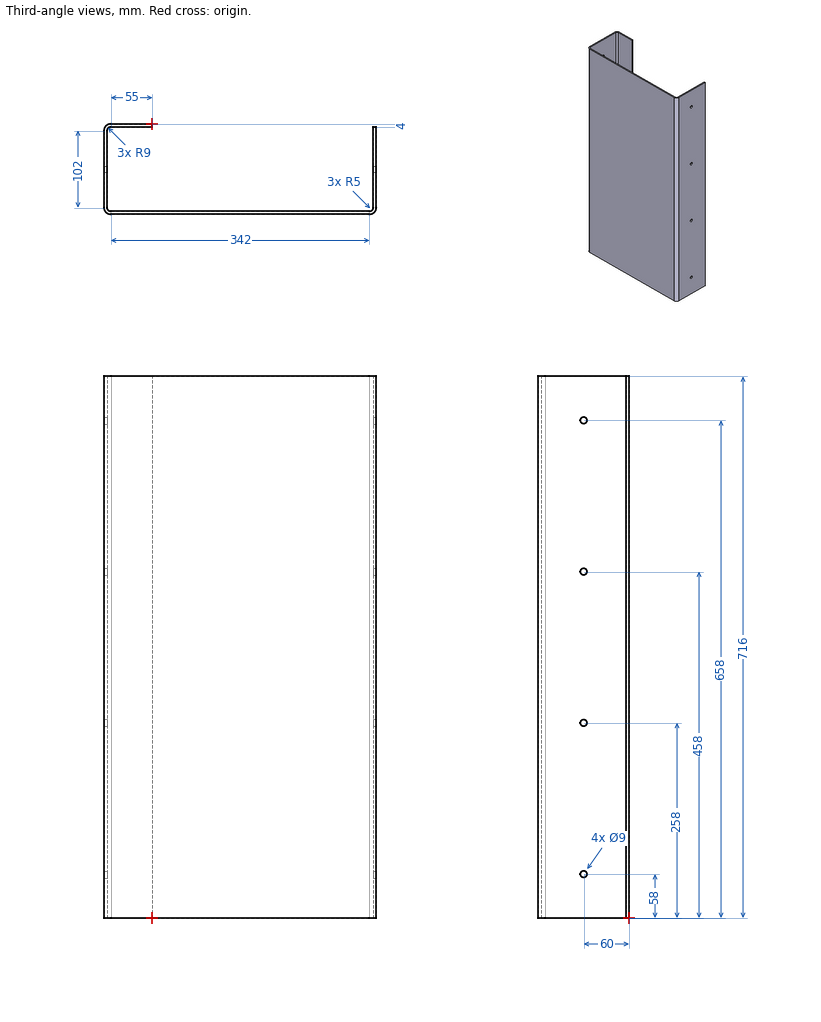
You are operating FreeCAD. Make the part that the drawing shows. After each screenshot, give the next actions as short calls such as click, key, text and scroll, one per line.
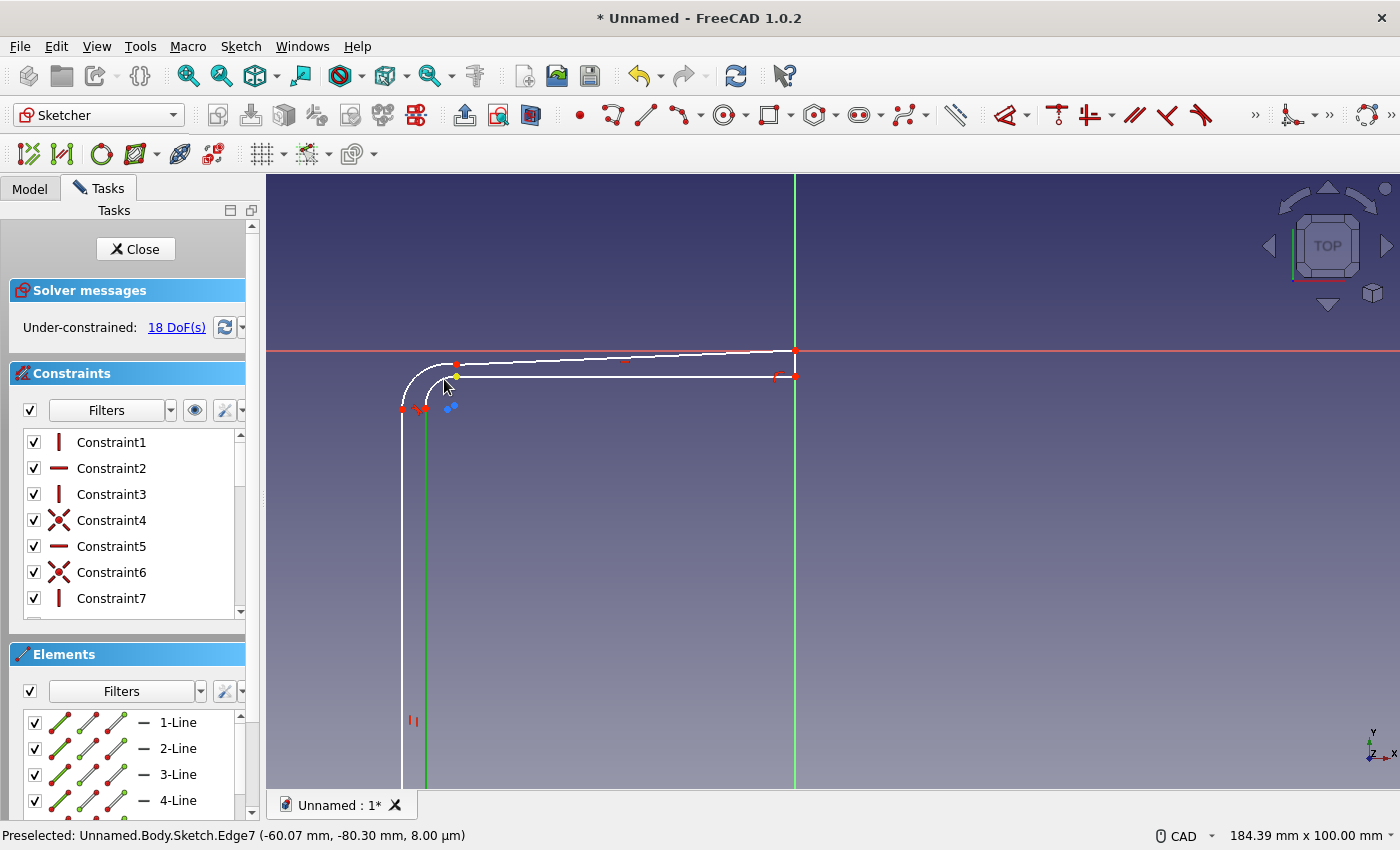
click(442, 380)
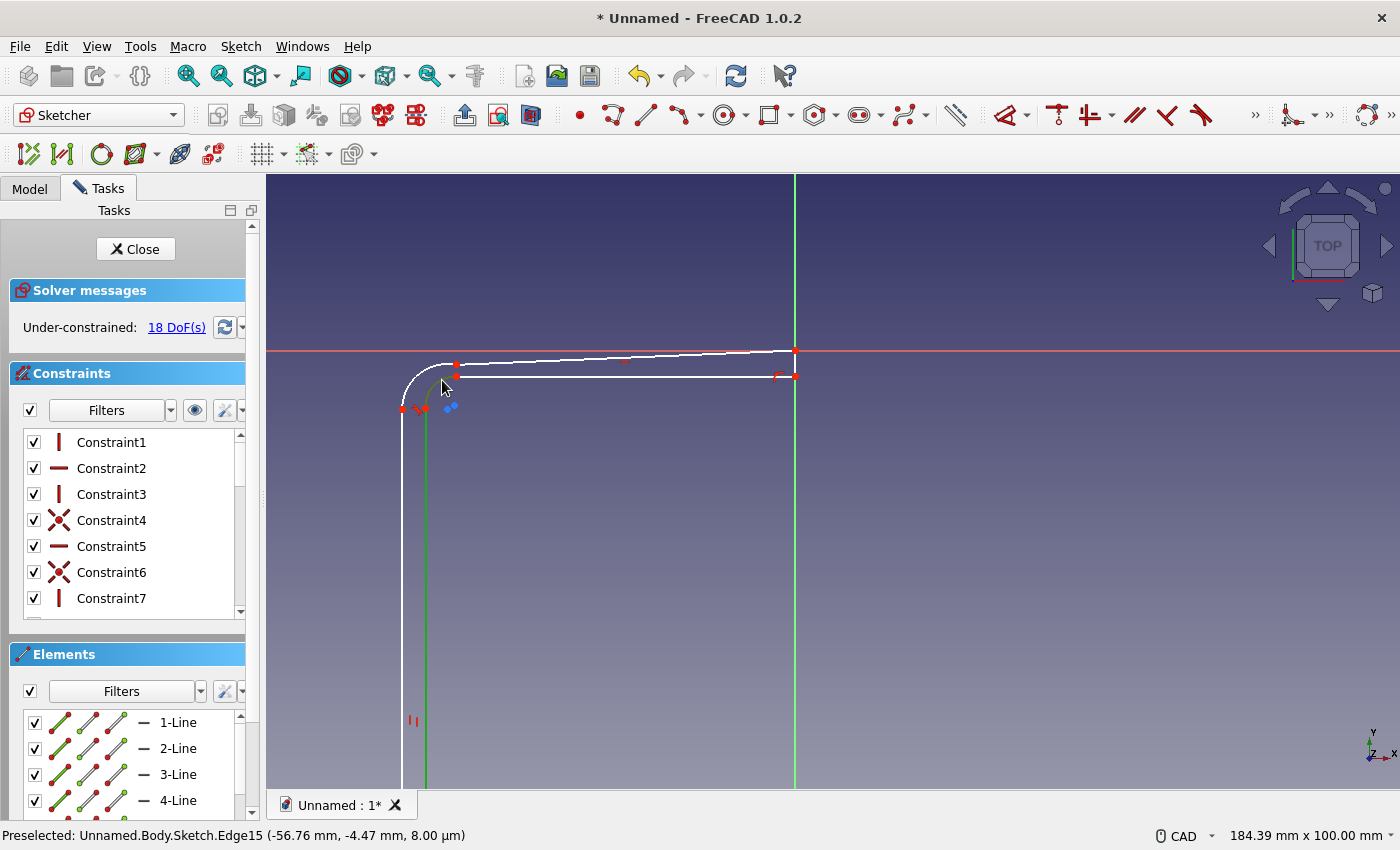
click(1201, 116)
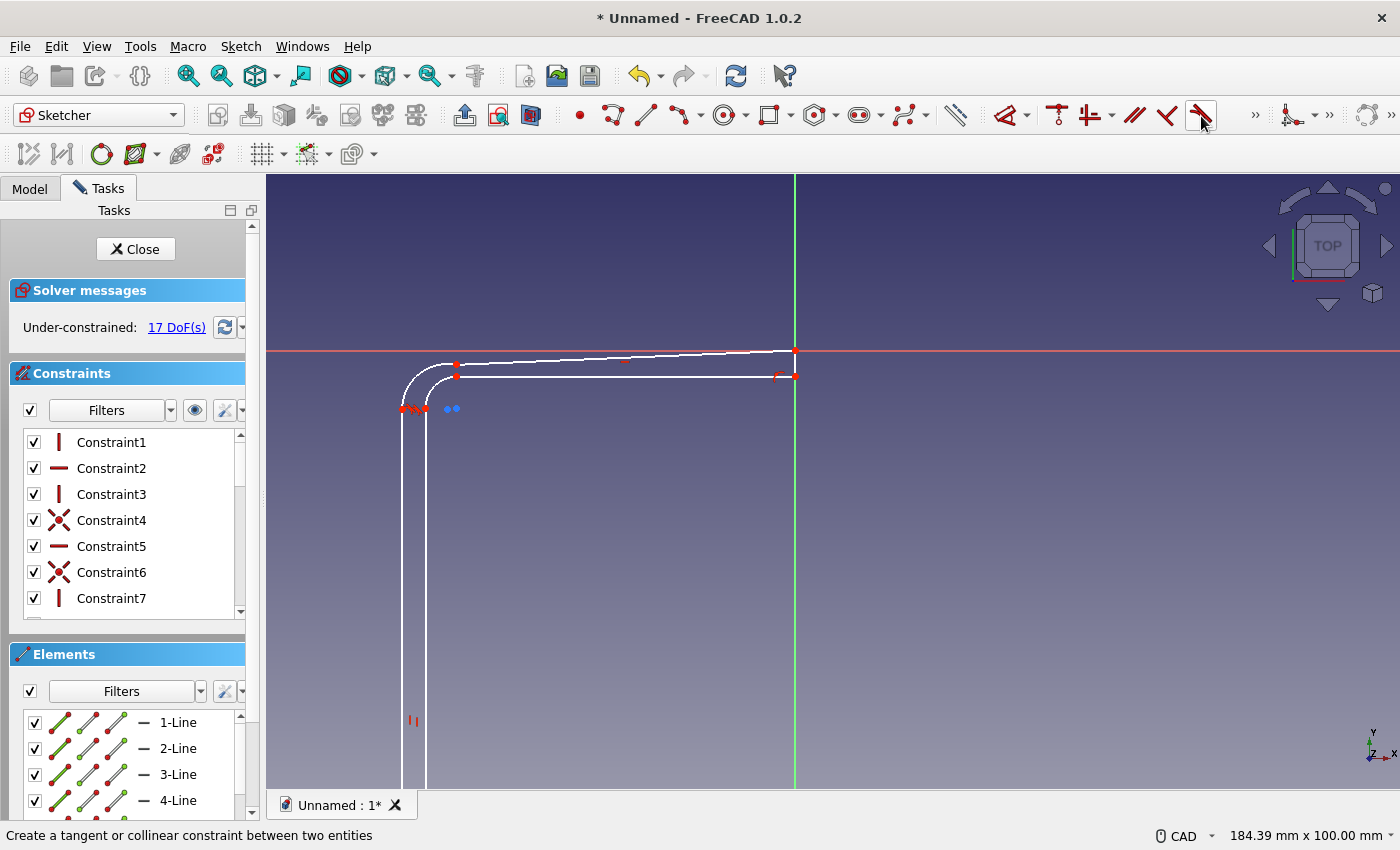
click(558, 377)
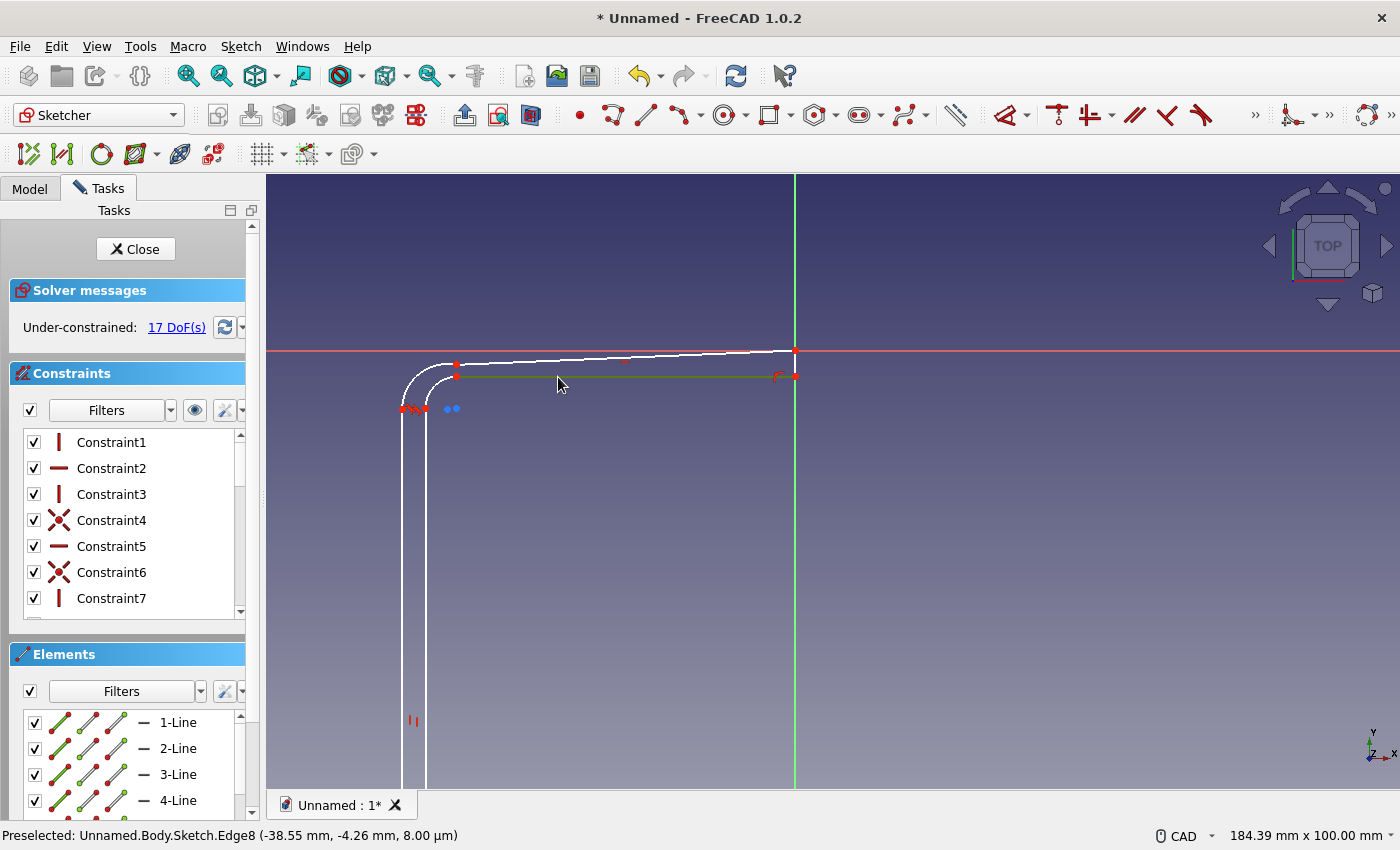
click(443, 380)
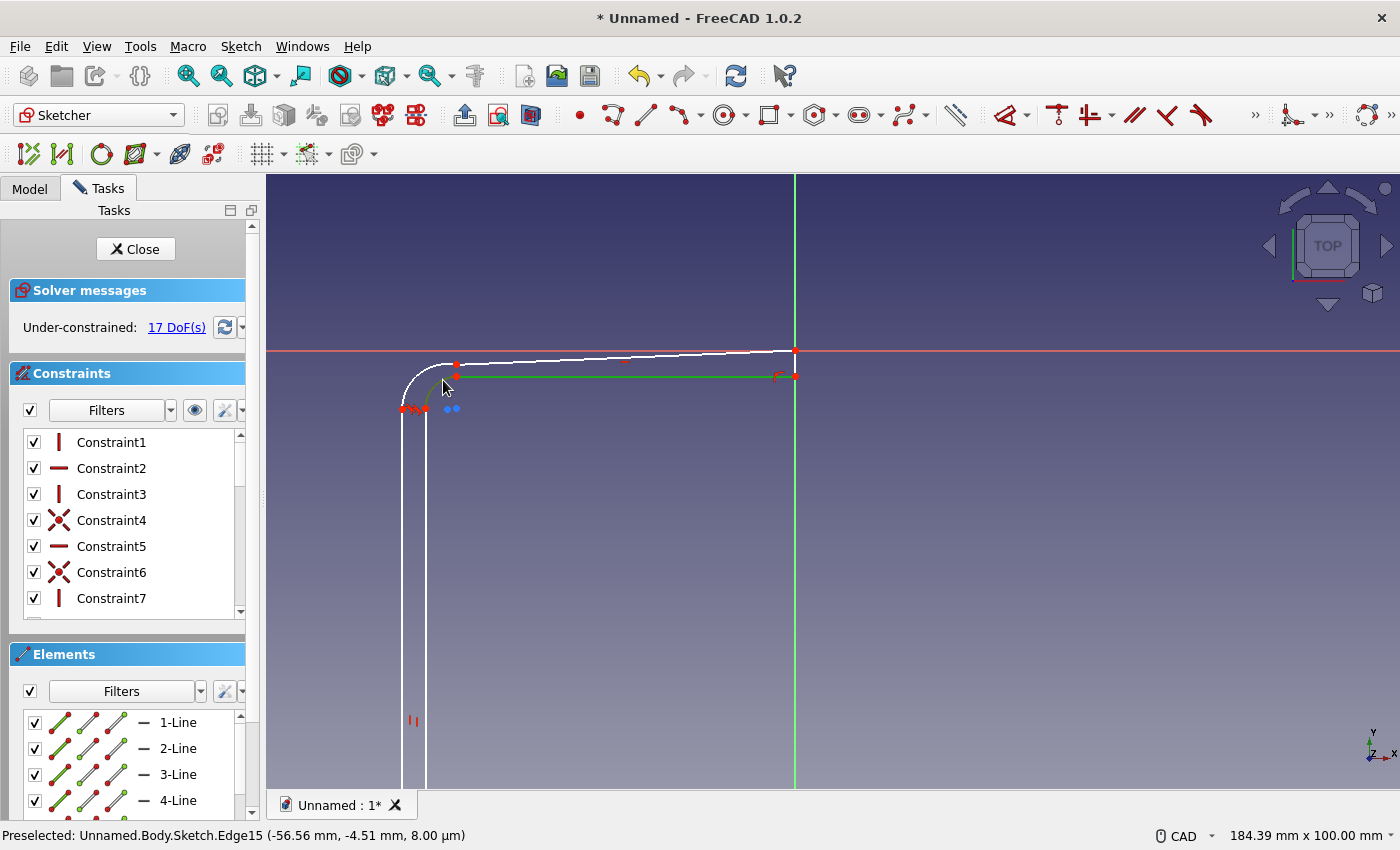
click(1201, 116)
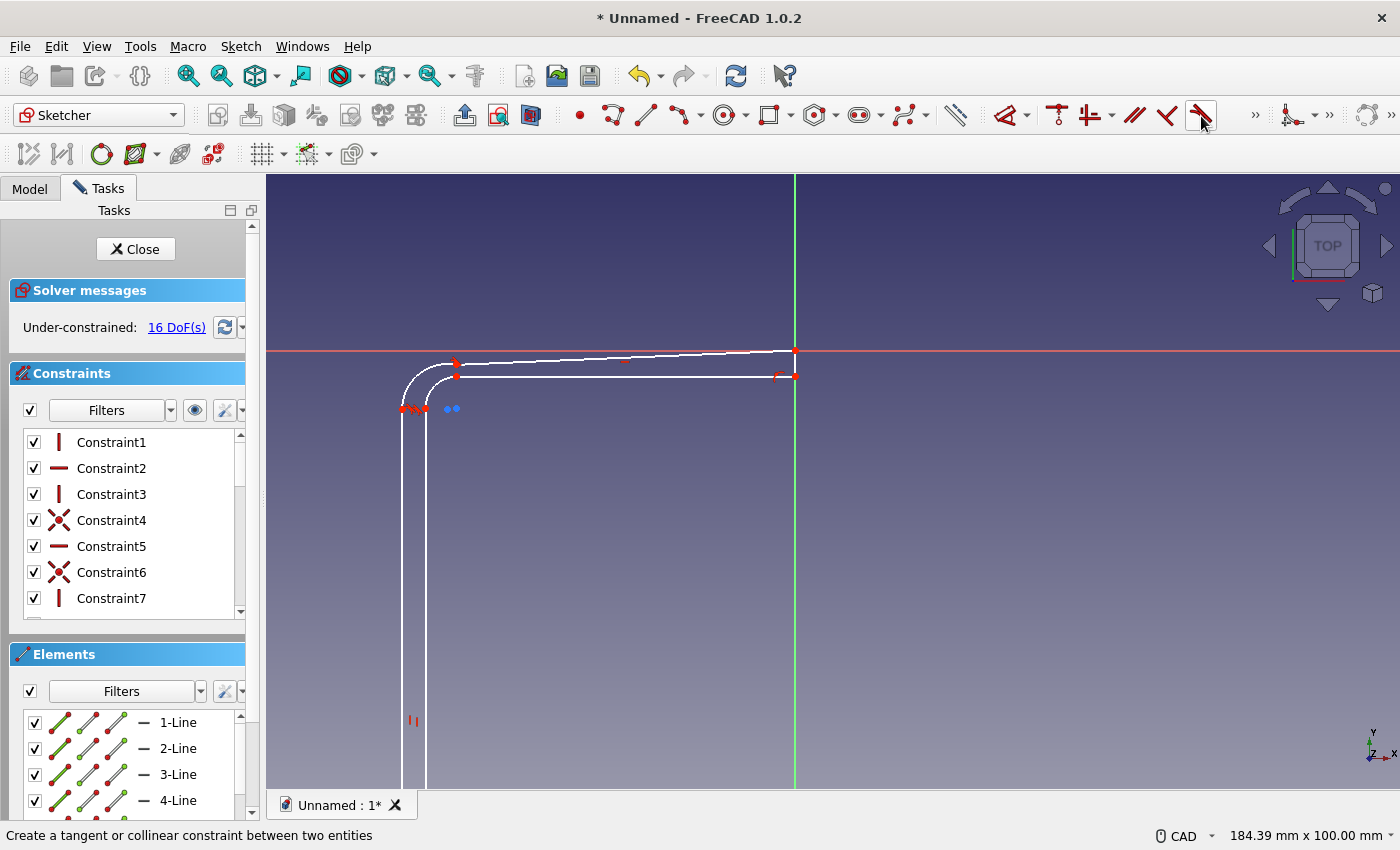
scroll(558, 361, up, 2)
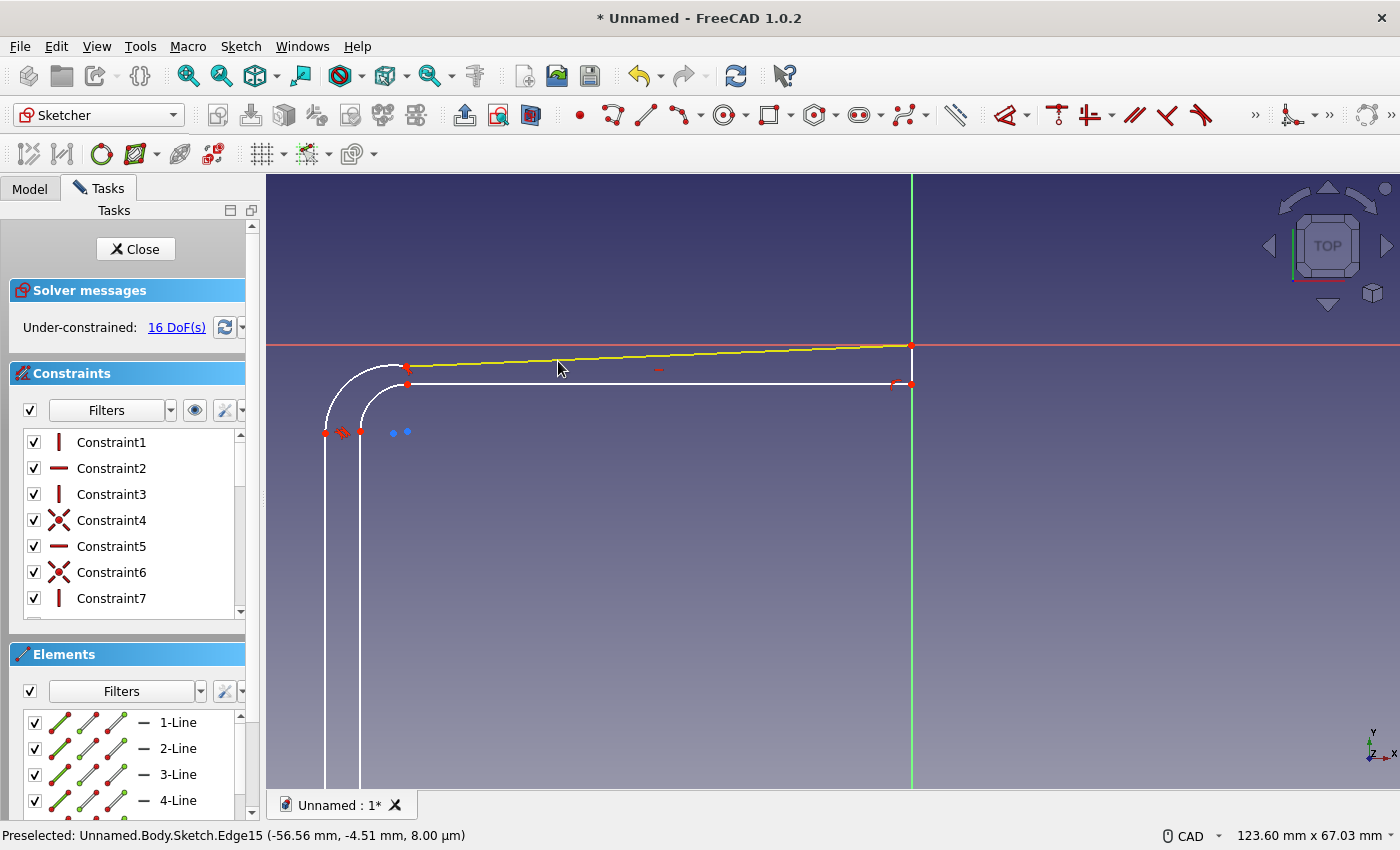
click(558, 360)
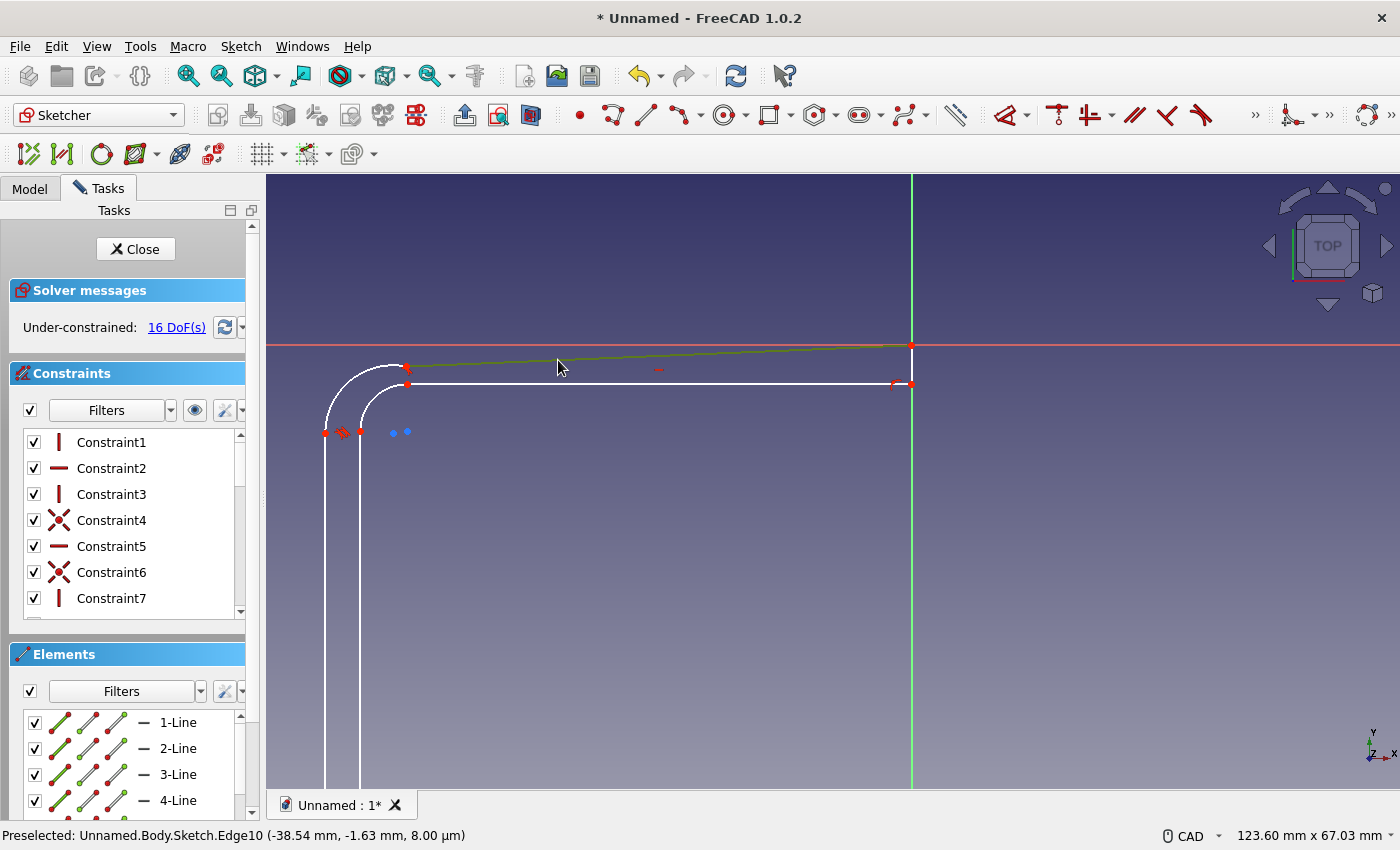
click(371, 369)